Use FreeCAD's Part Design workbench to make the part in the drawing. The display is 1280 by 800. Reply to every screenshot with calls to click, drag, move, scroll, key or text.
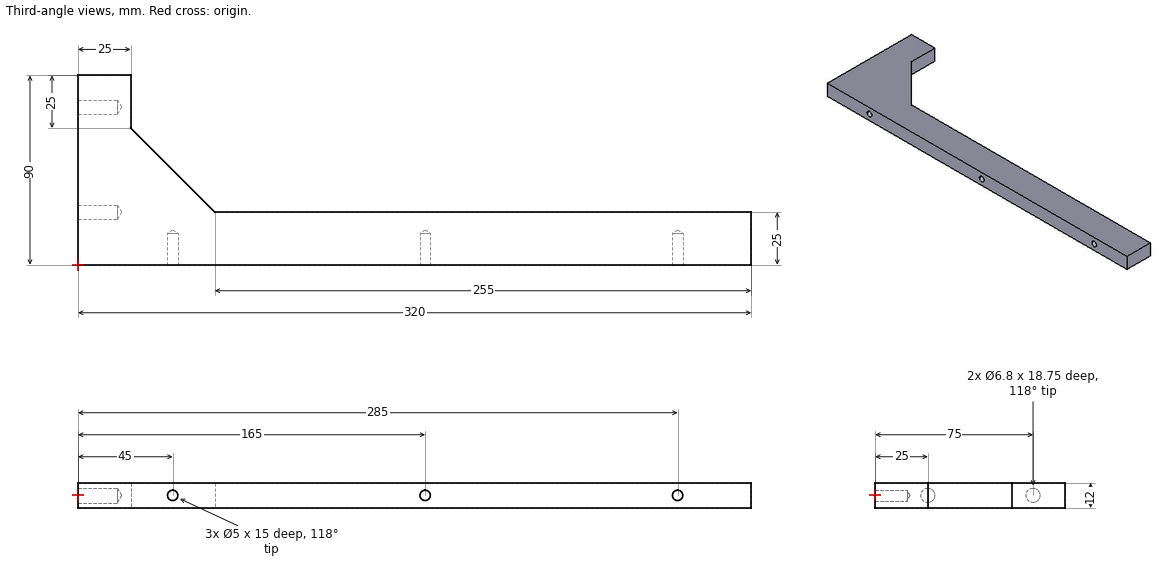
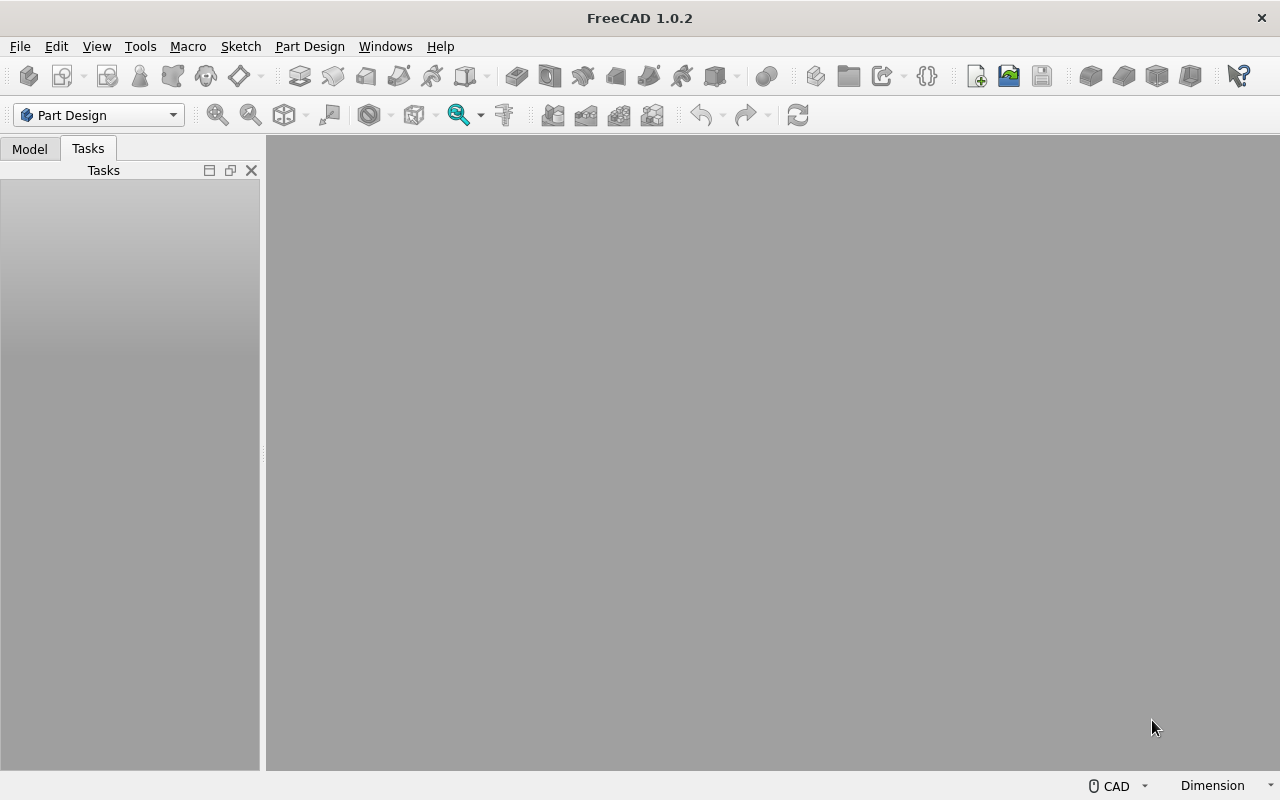
key(ctrl+n)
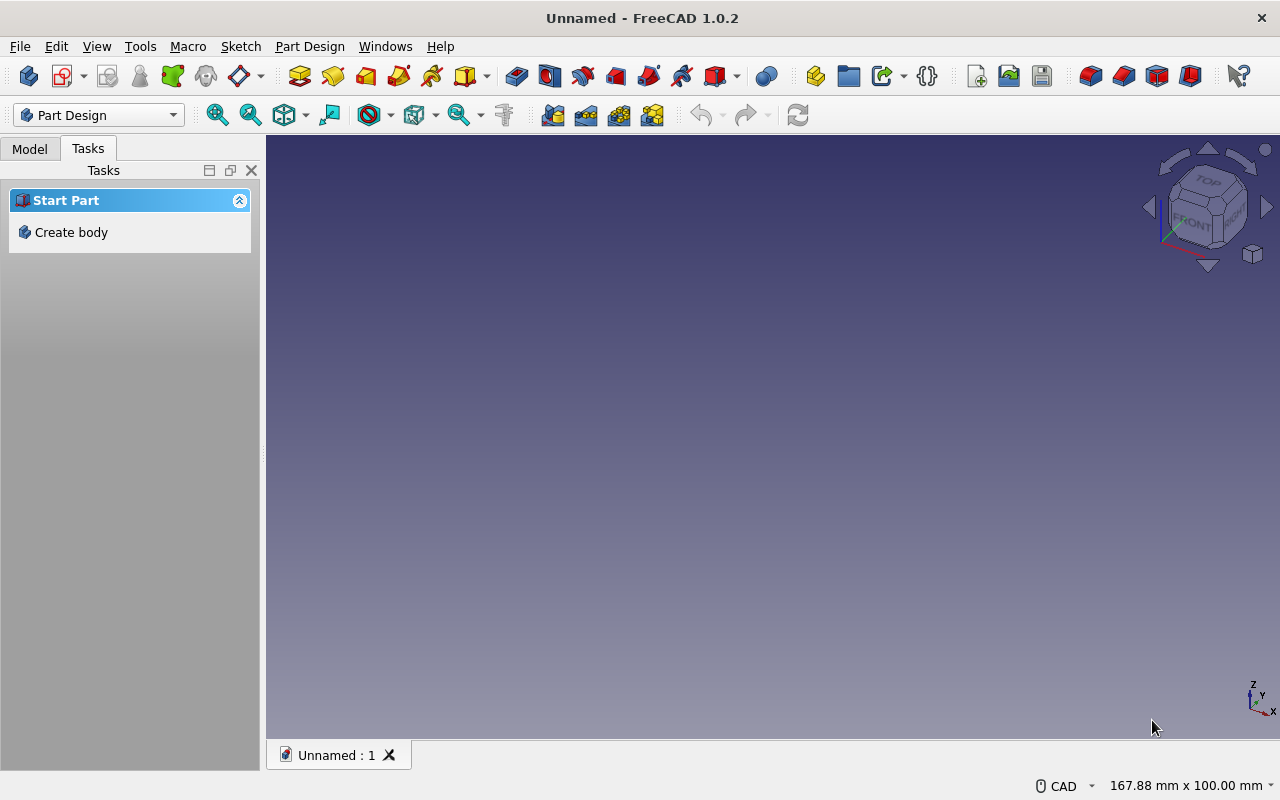
click(62, 76)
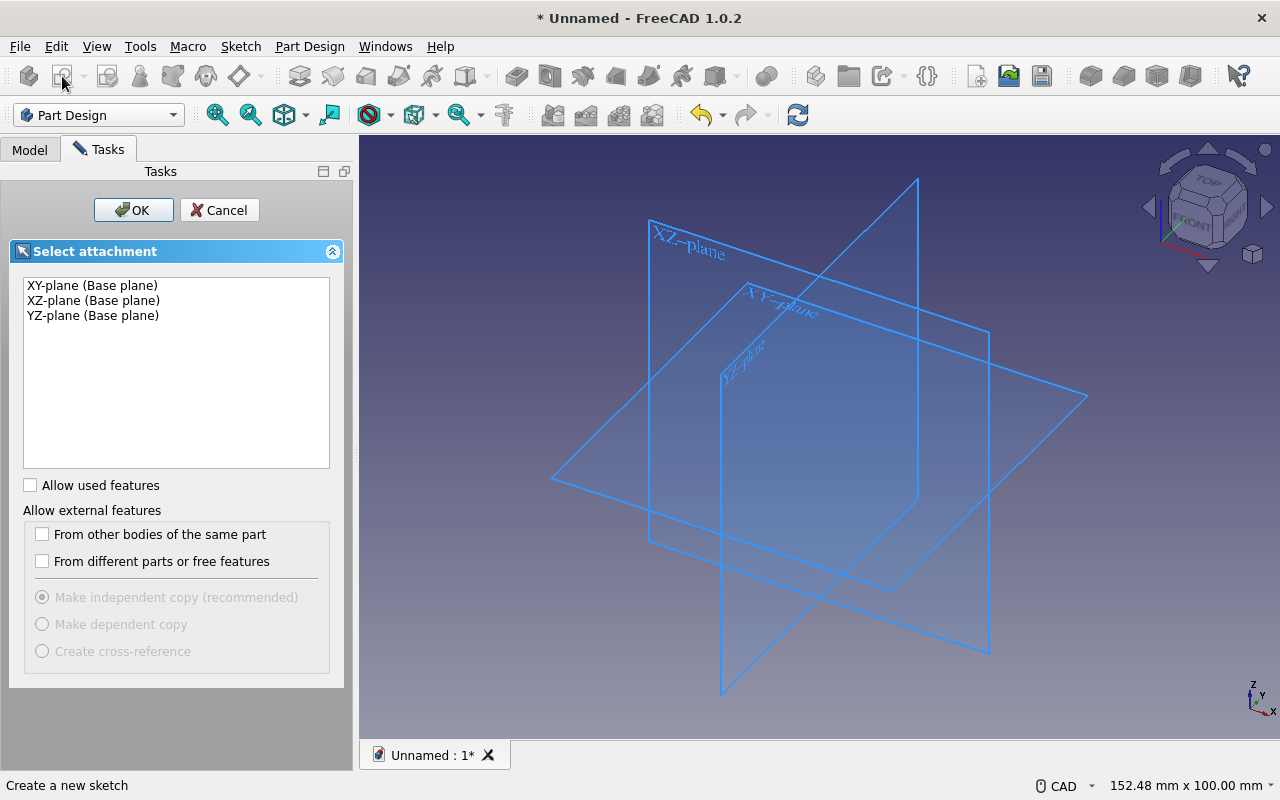
click(84, 286)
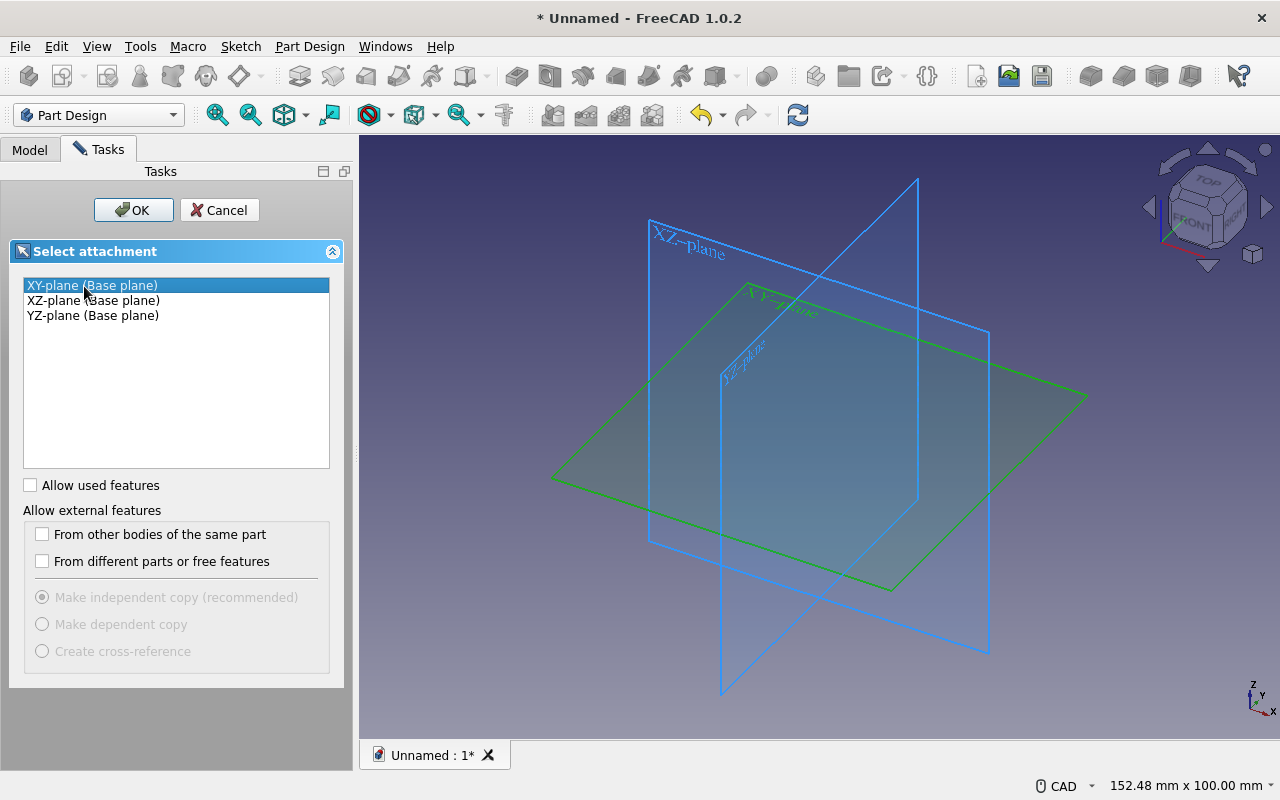
click(134, 210)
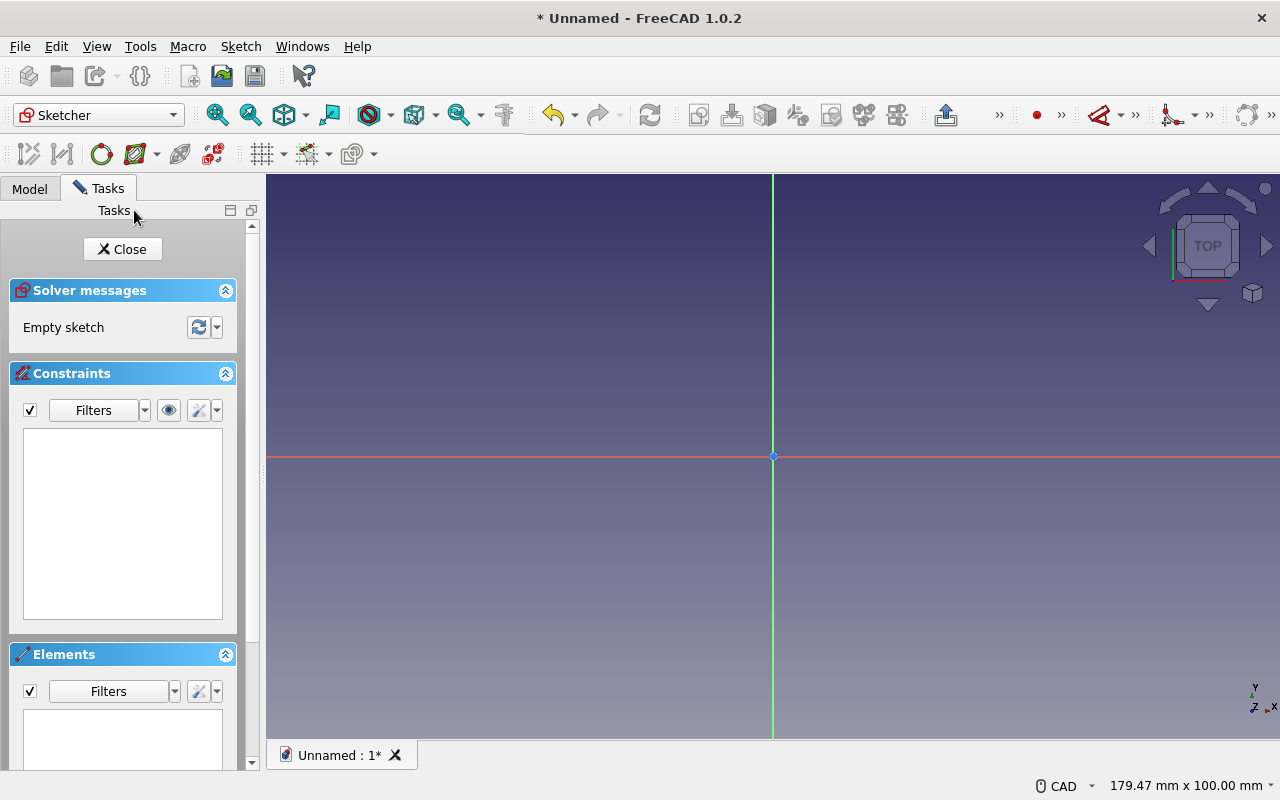
scroll(294, 566, down, 6)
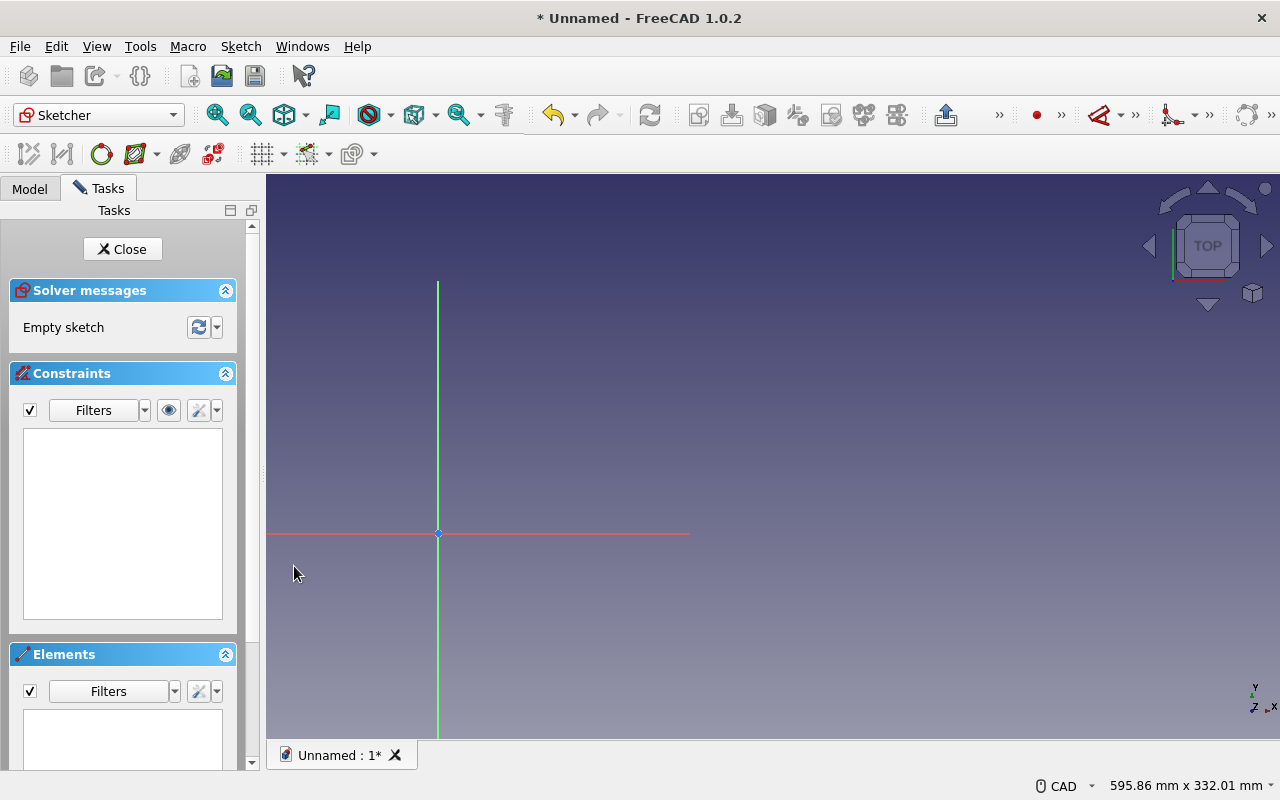
key(g)
key(m)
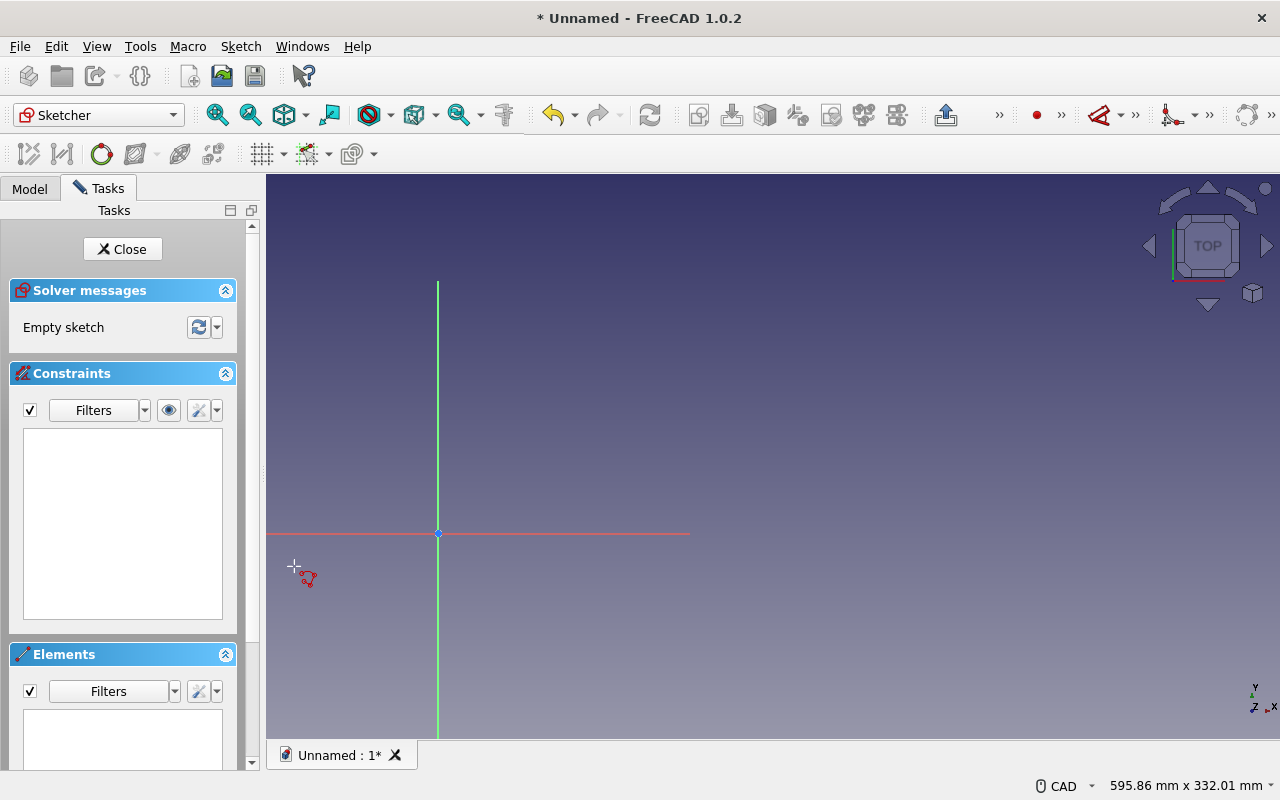
click(438, 534)
click(983, 525)
click(983, 491)
click(549, 491)
click(481, 423)
click(481, 380)
click(447, 380)
click(438, 534)
key(Escape)
key(Escape)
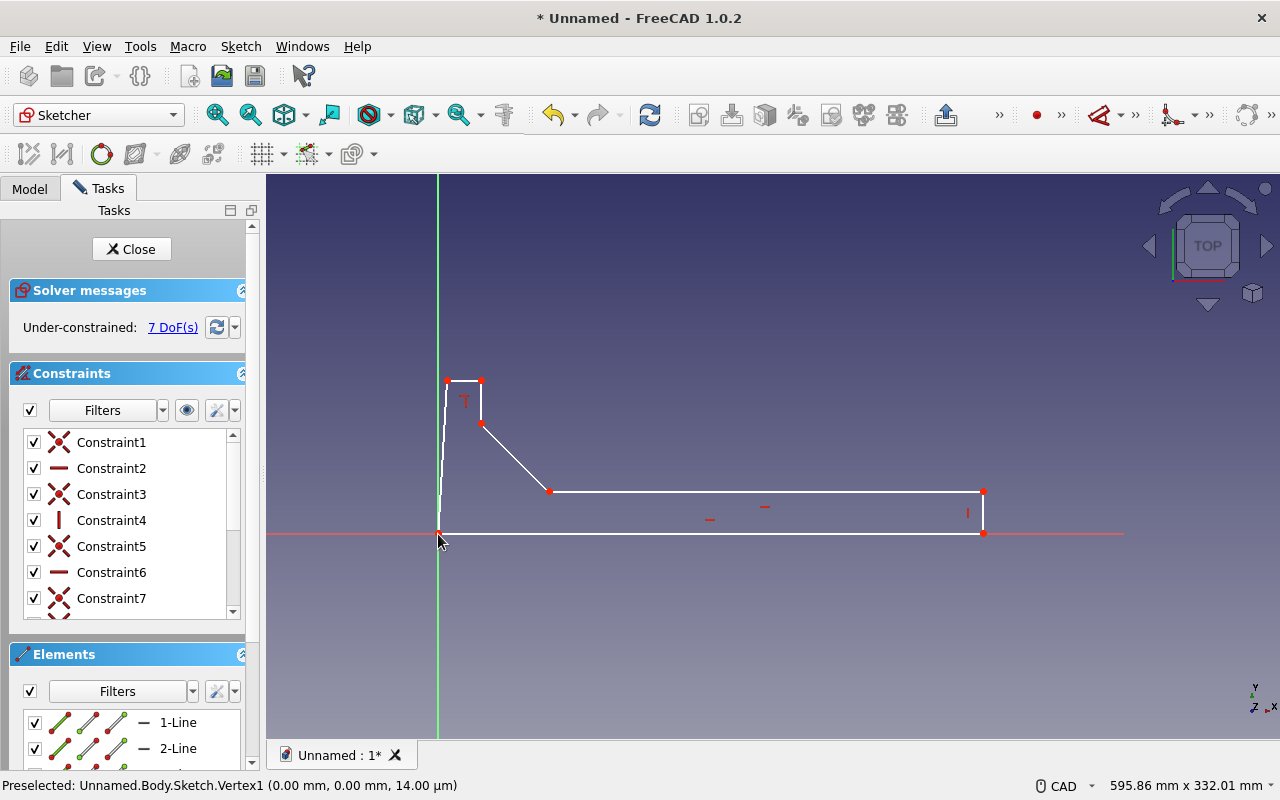
click(441, 488)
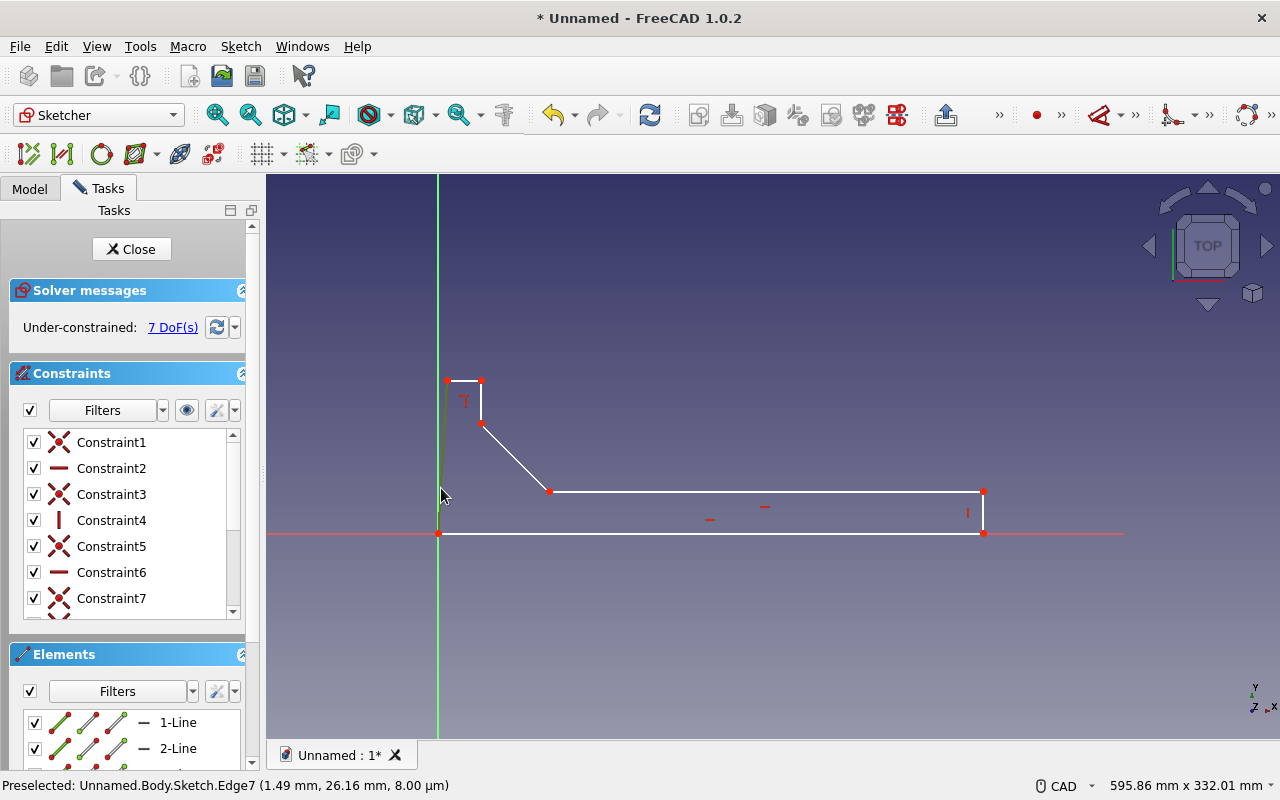
key(v)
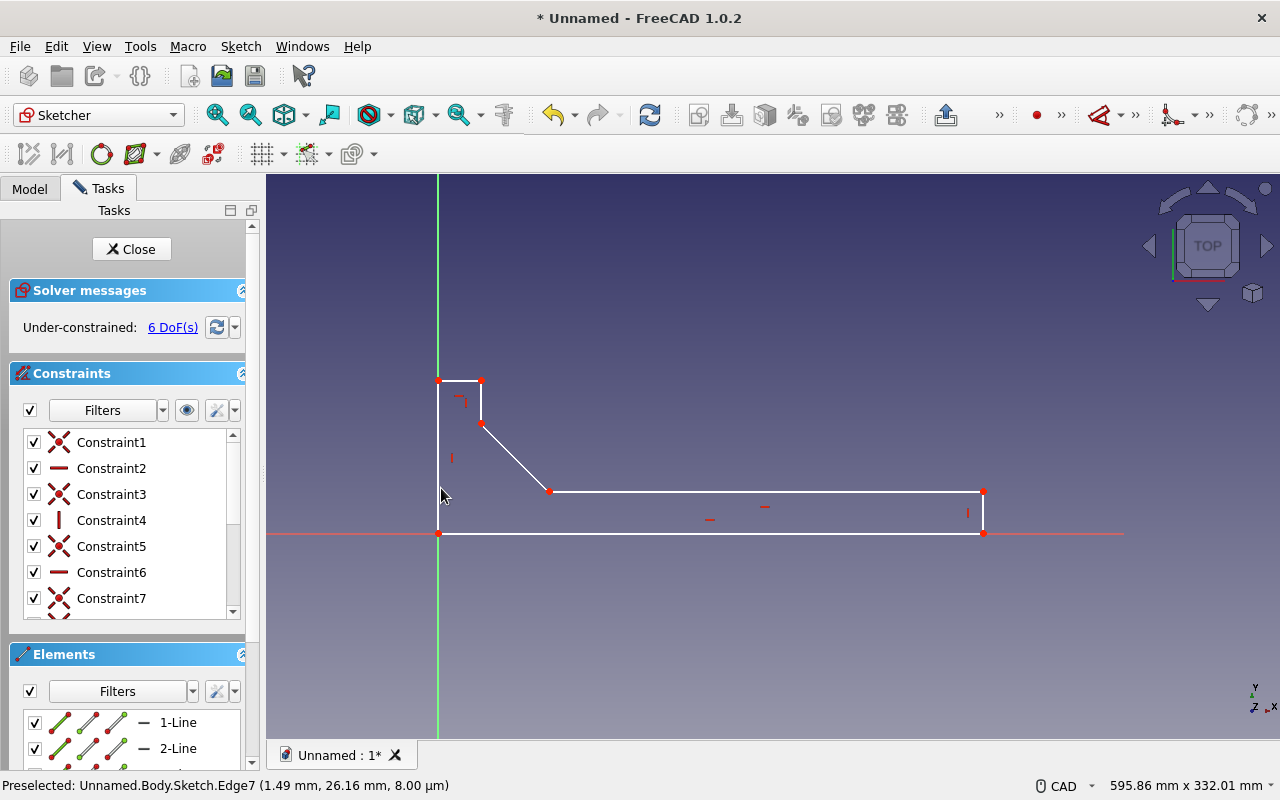
key(d)